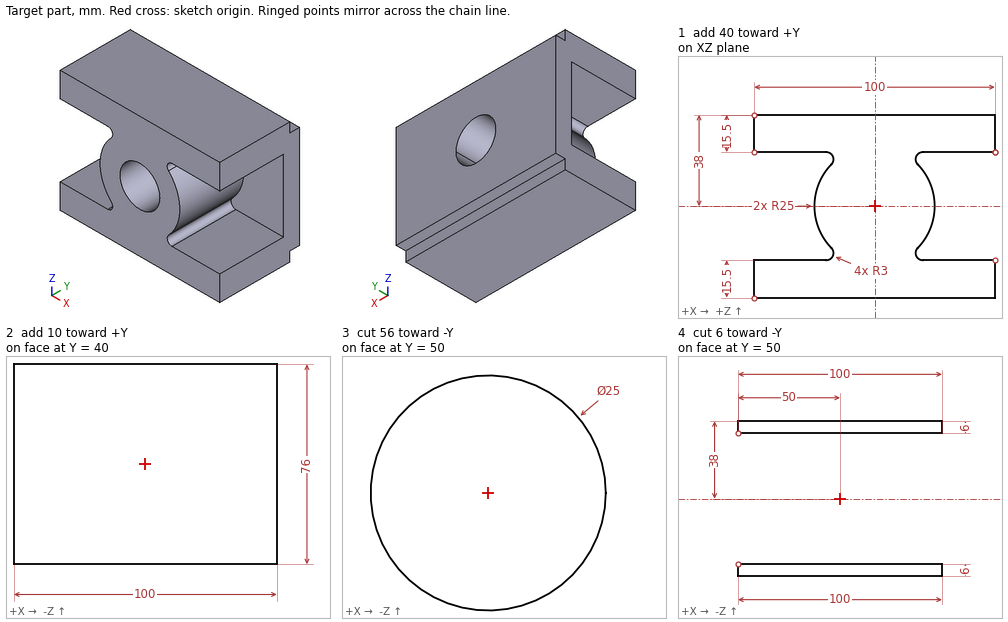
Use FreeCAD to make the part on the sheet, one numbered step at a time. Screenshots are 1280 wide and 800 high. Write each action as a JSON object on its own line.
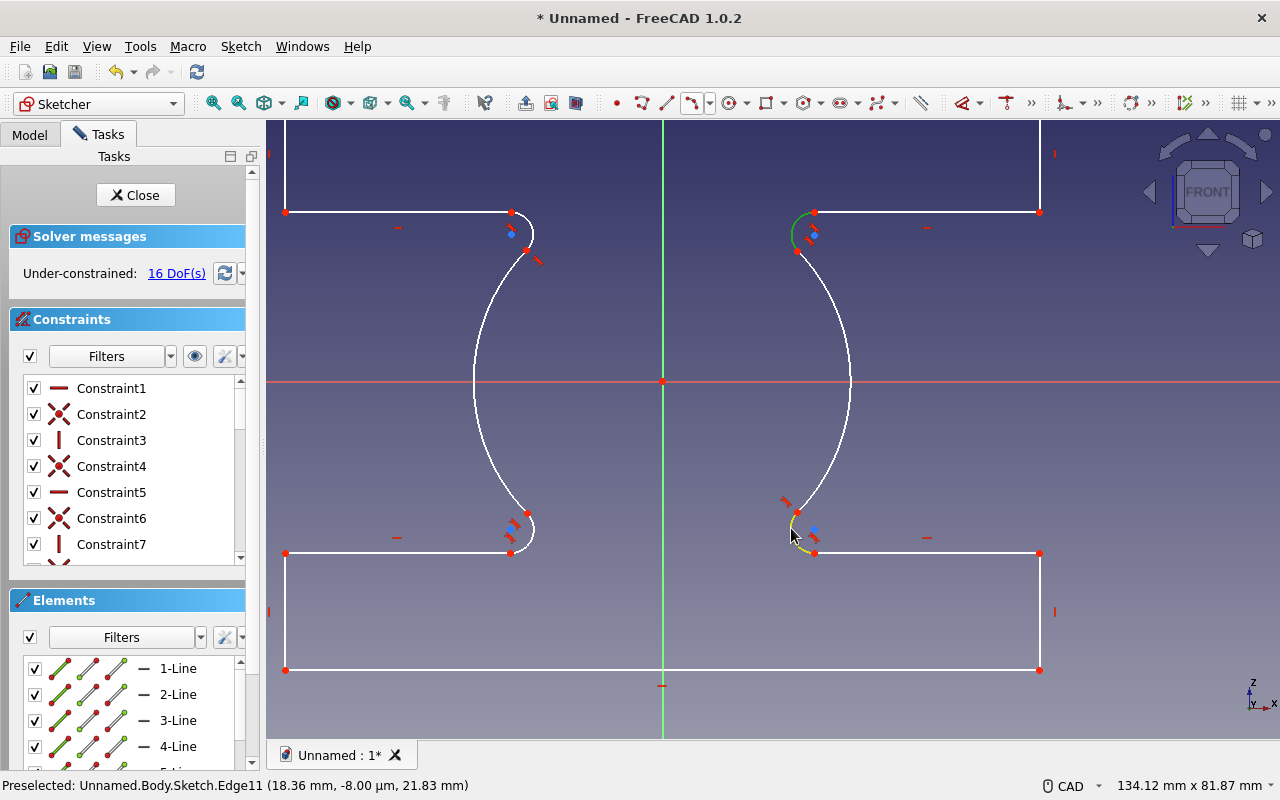
{"action": "left_click", "coordinate": [791, 528]}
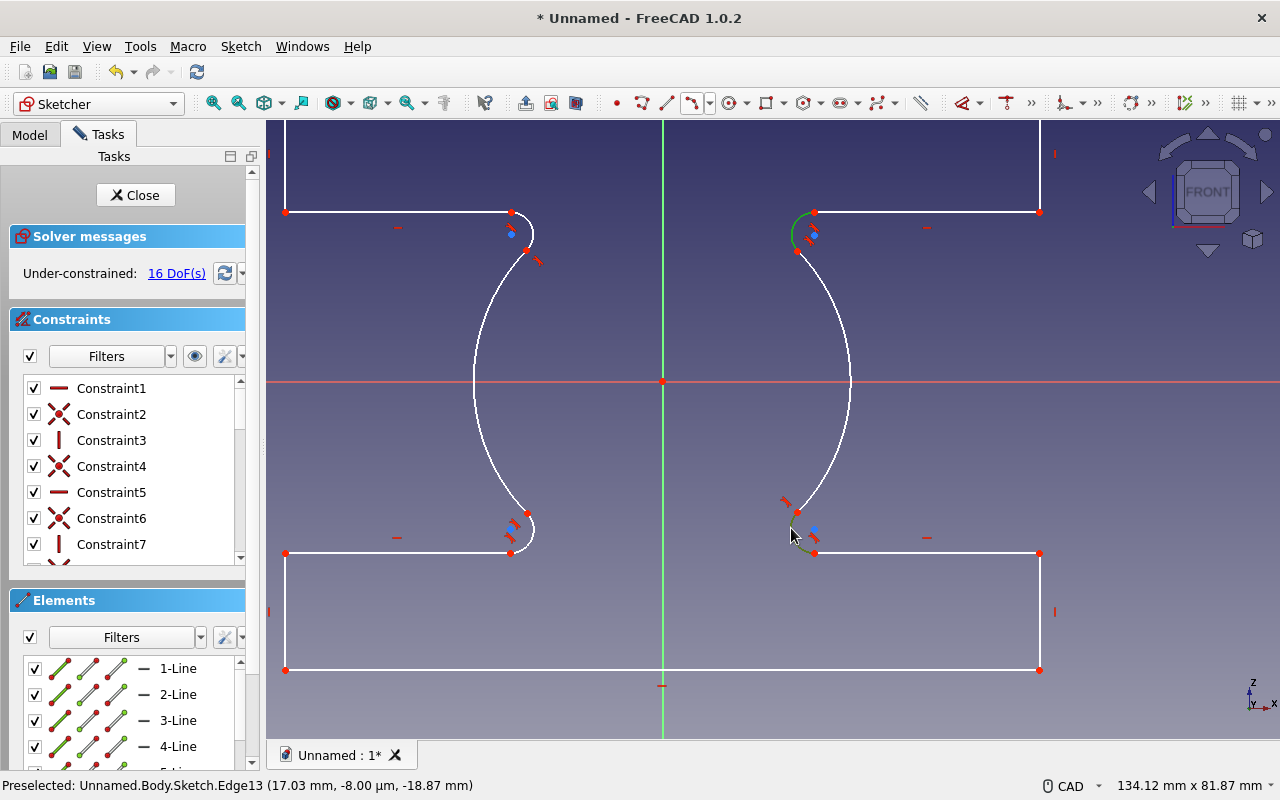
{"action": "left_click", "coordinate": [525, 548]}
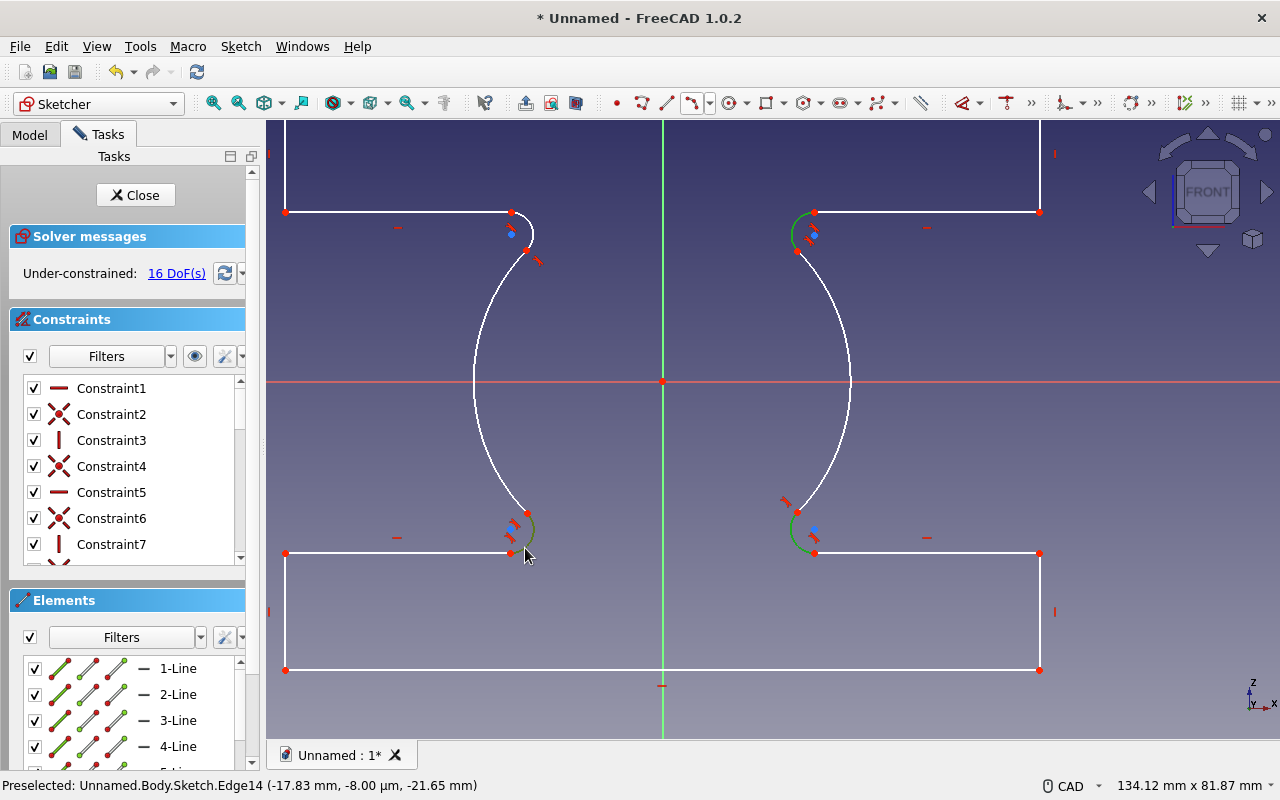
{"action": "left_click", "coordinate": [533, 236]}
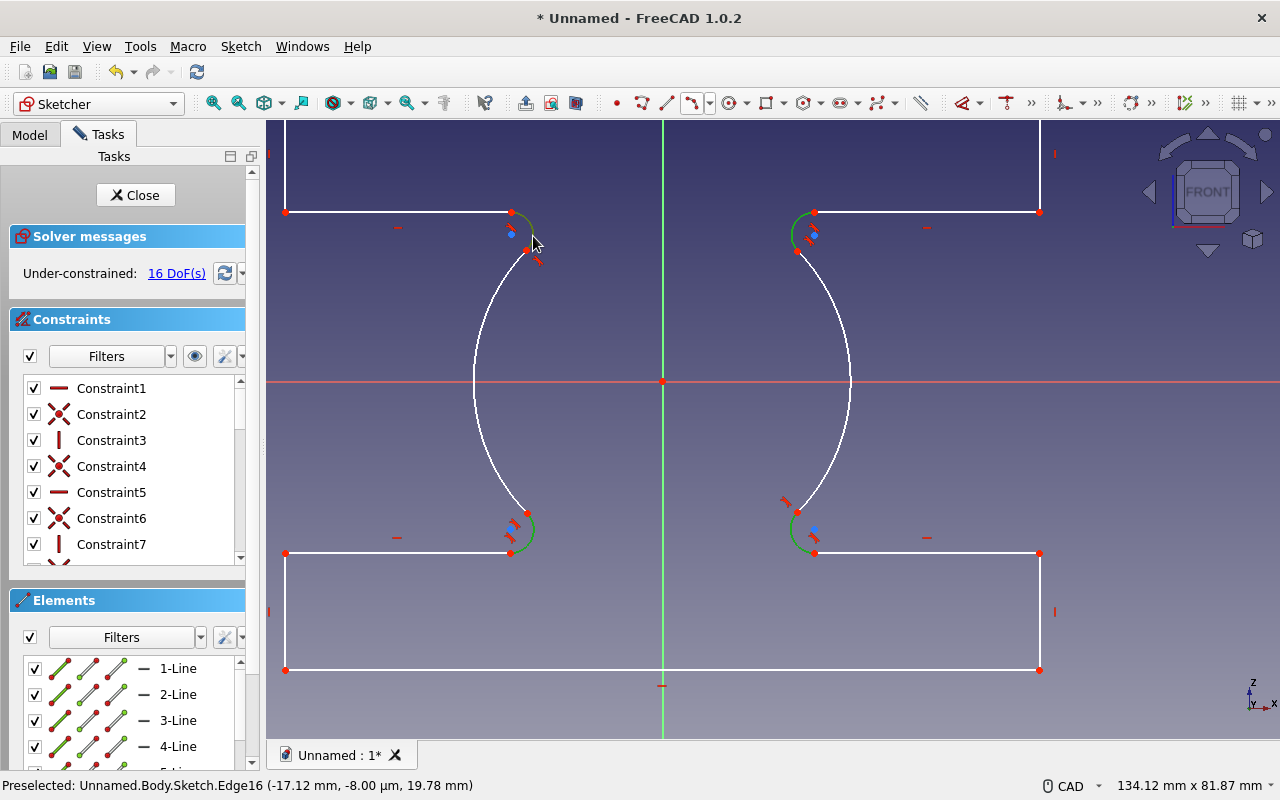
{"action": "key", "text": "e"}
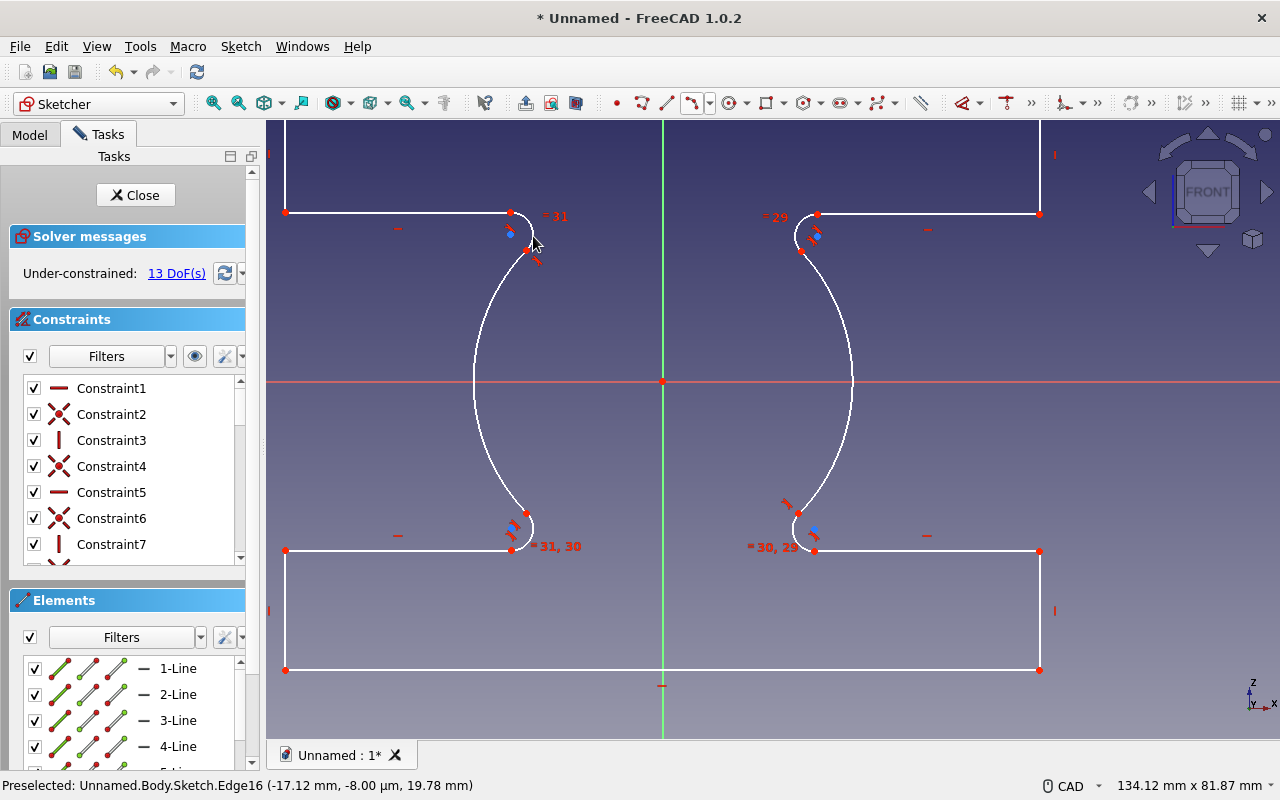
{"action": "left_click", "coordinate": [843, 440]}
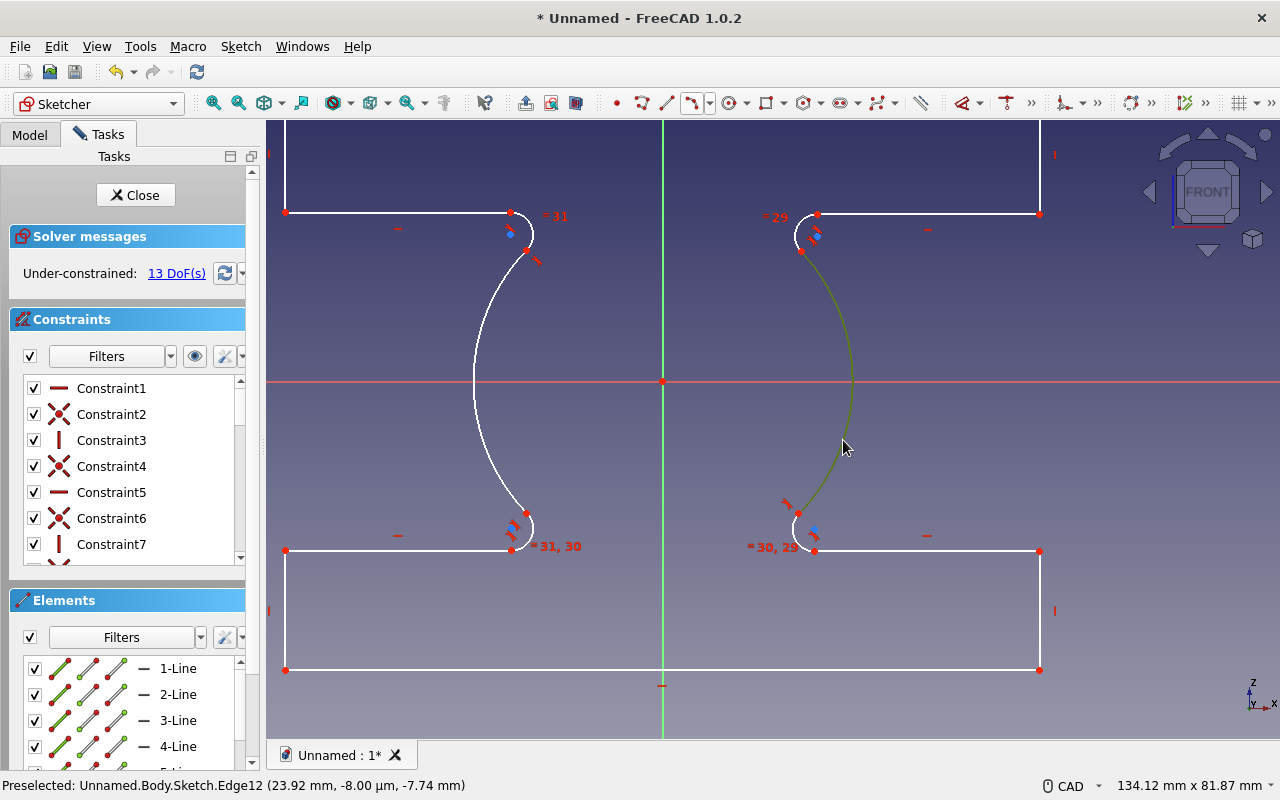
{"action": "left_click", "coordinate": [482, 324]}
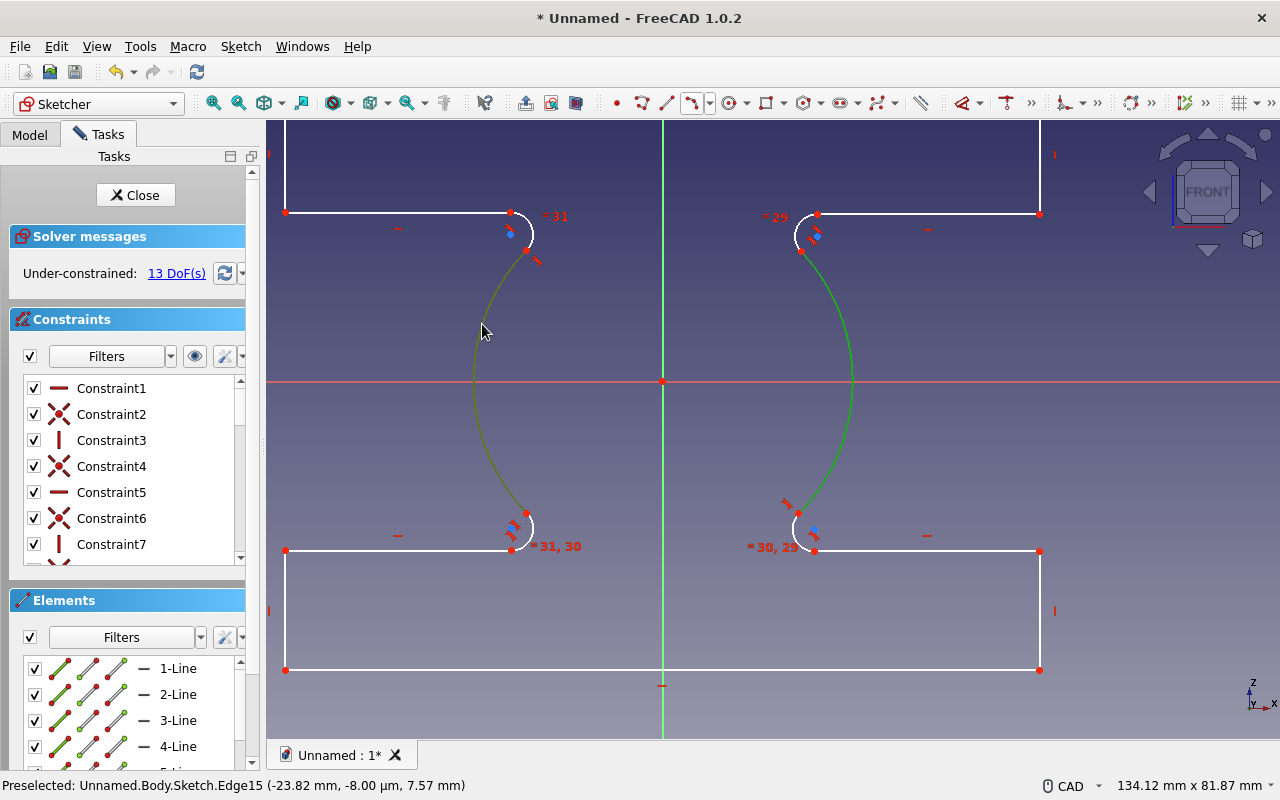
{"action": "key", "text": "e"}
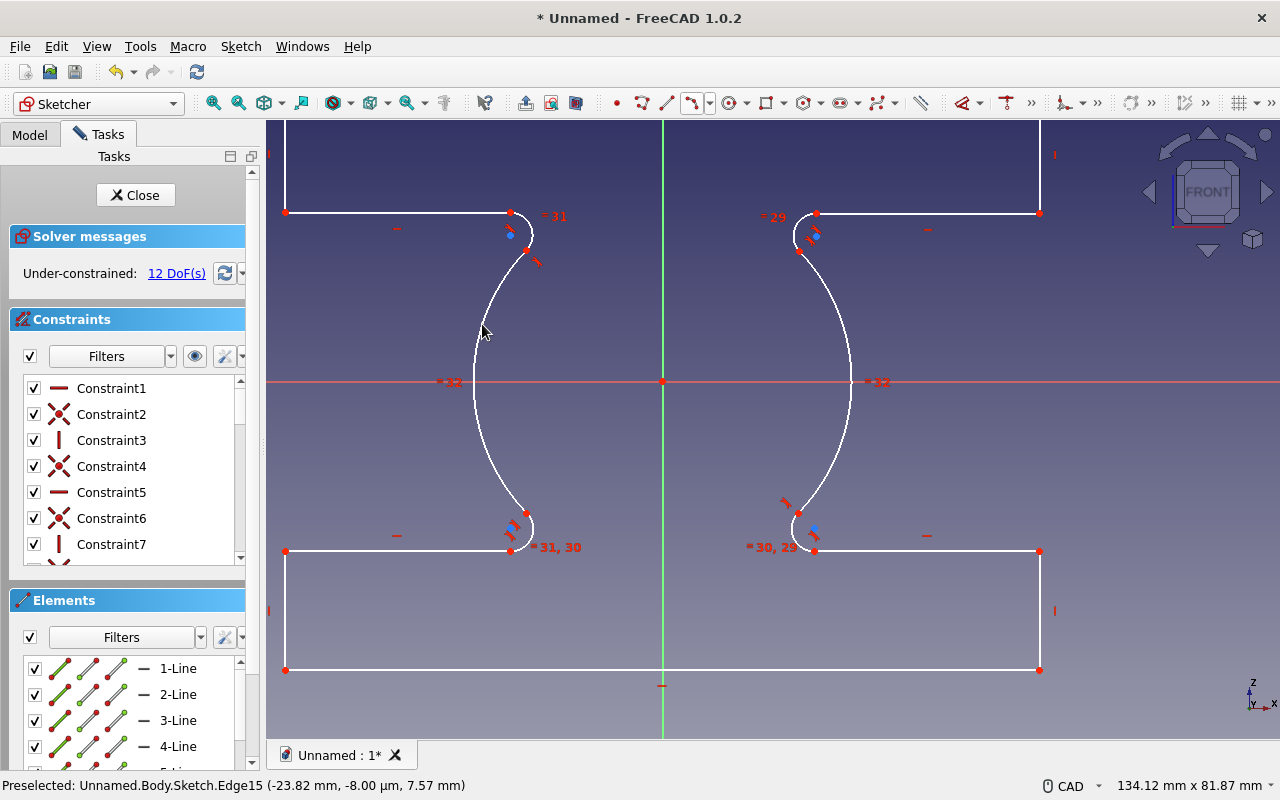
{"action": "scroll", "coordinate": [790, 527], "scroll_direction": "down", "scroll_amount": 2}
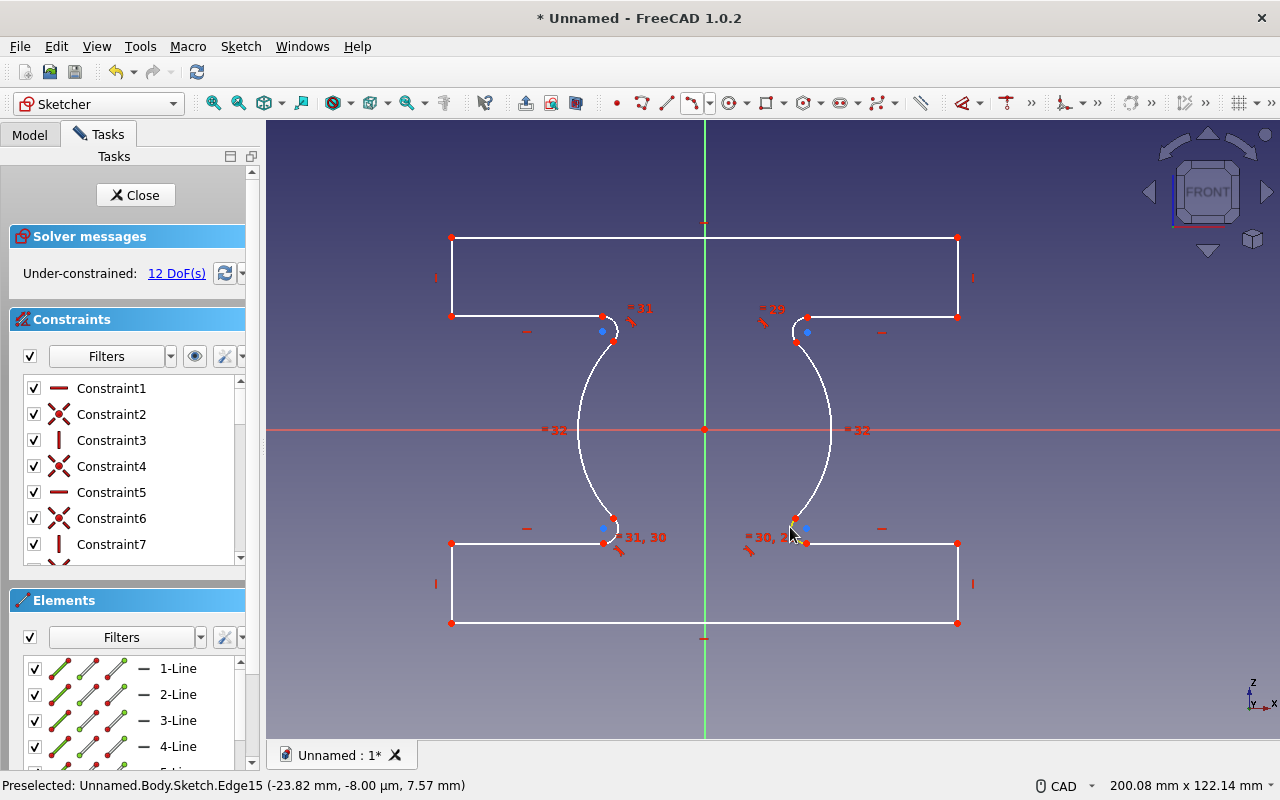
{"action": "left_click", "coordinate": [452, 316]}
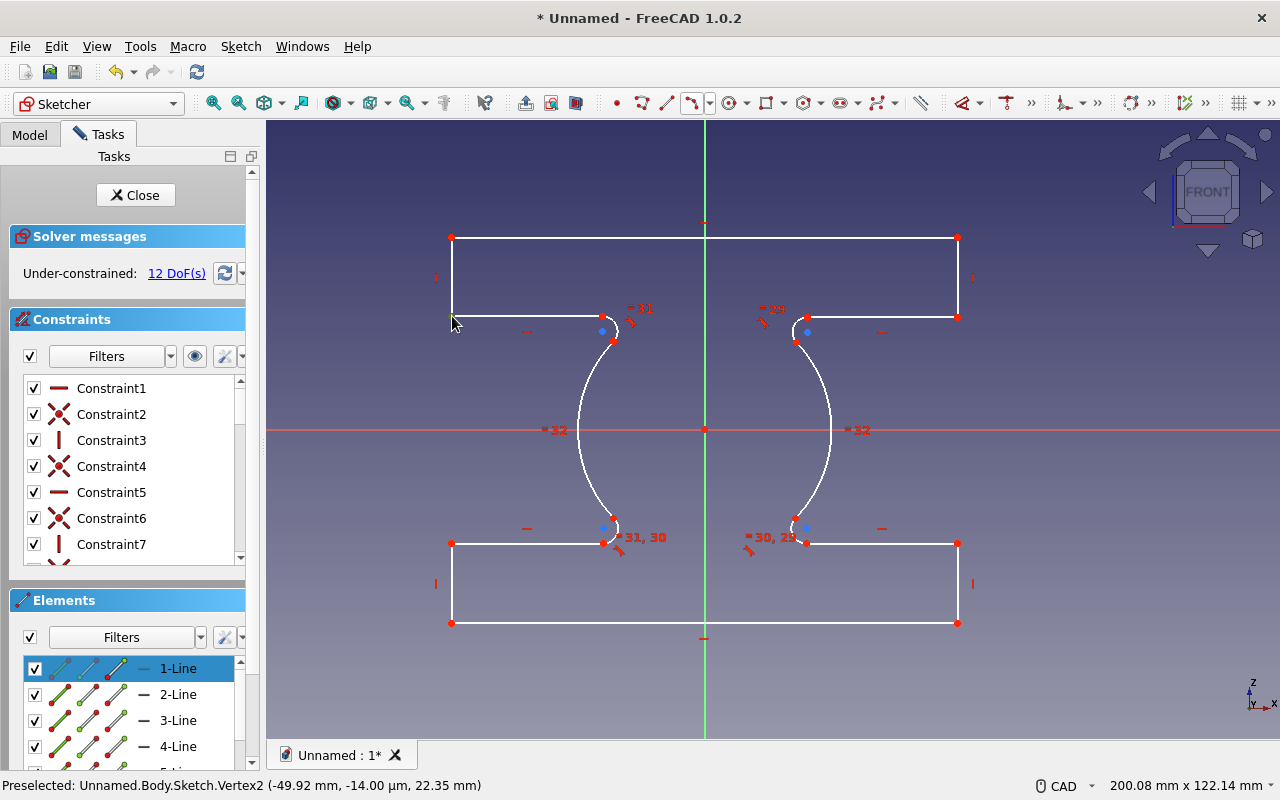
{"action": "left_click", "coordinate": [958, 317]}